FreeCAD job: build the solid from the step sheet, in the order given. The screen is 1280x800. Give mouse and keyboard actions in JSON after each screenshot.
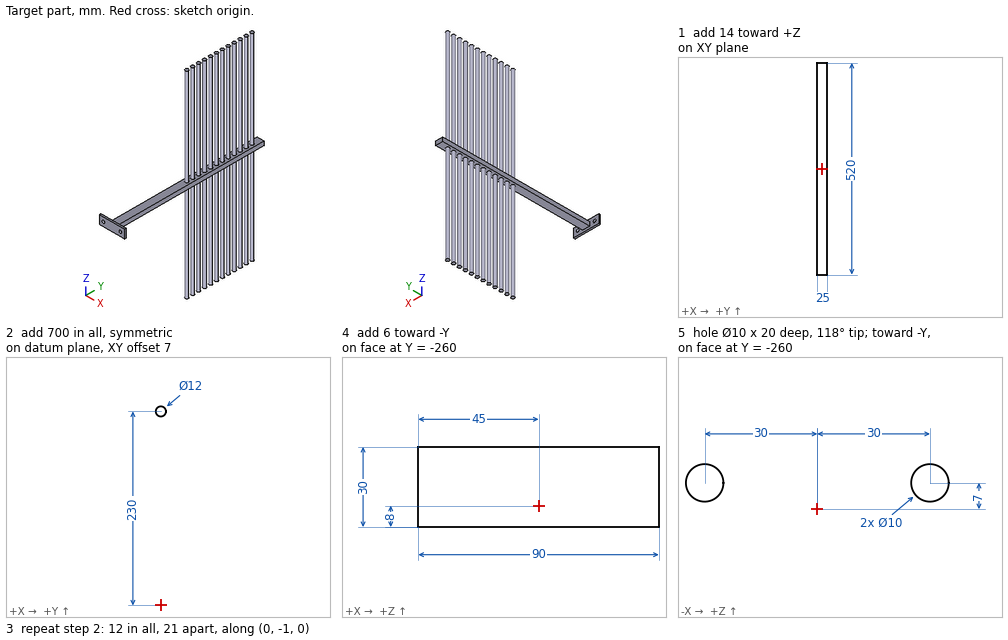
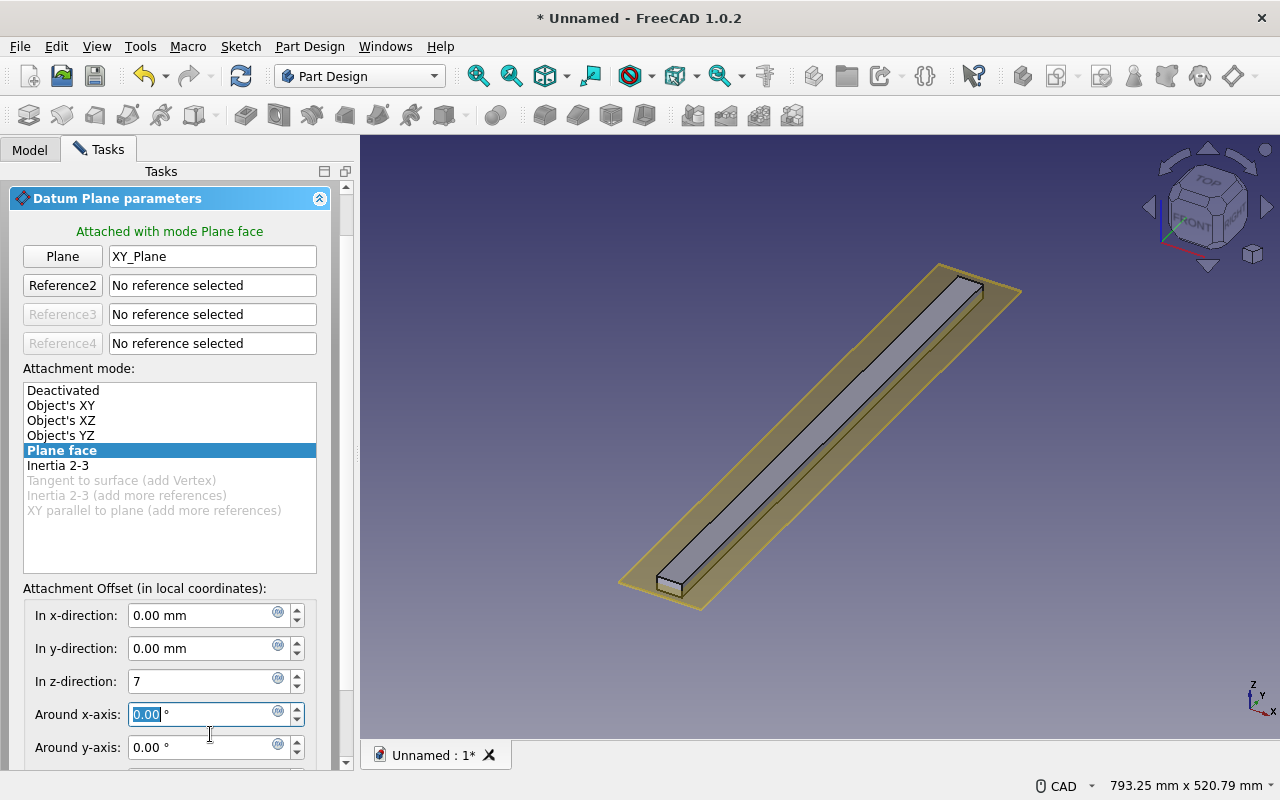
{"action": "scroll", "coordinate": [346, 476], "scroll_direction": "up", "scroll_amount": 2}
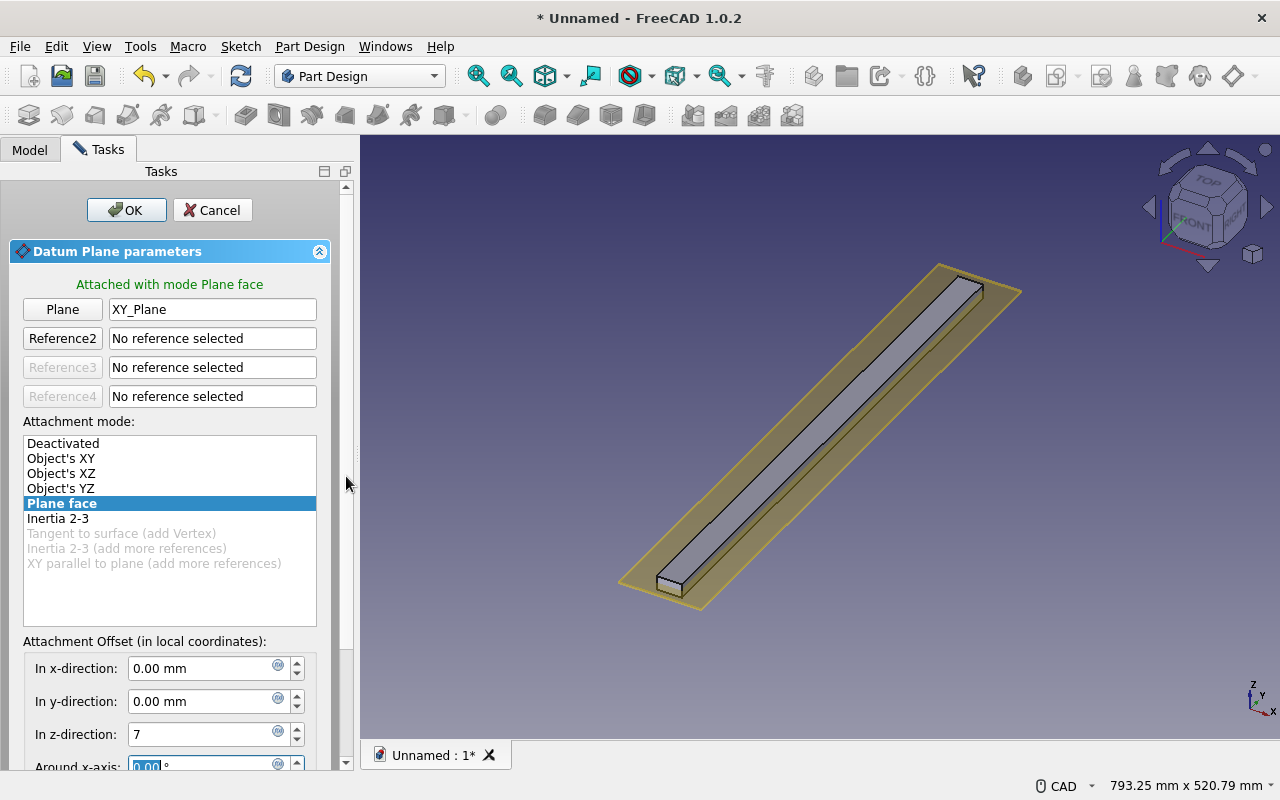
{"action": "left_click", "coordinate": [127, 210]}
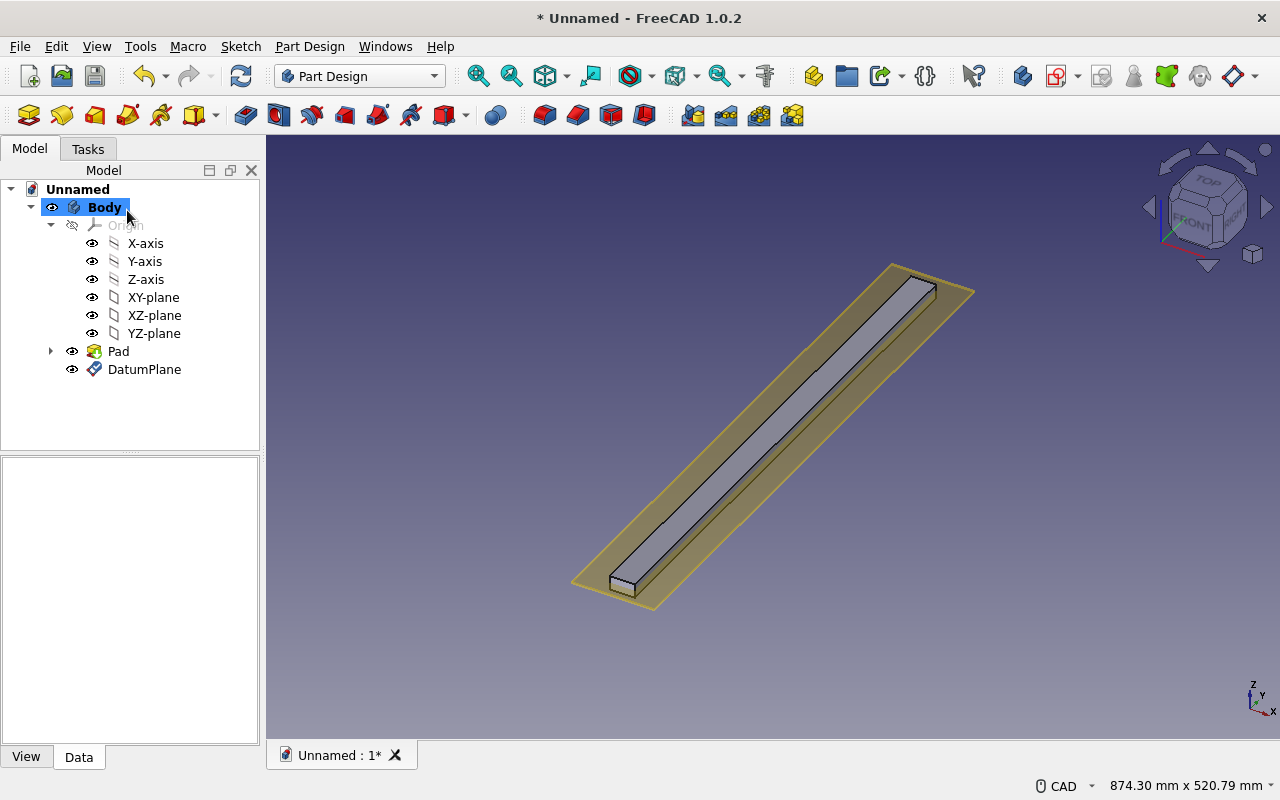
{"action": "left_click", "coordinate": [117, 369]}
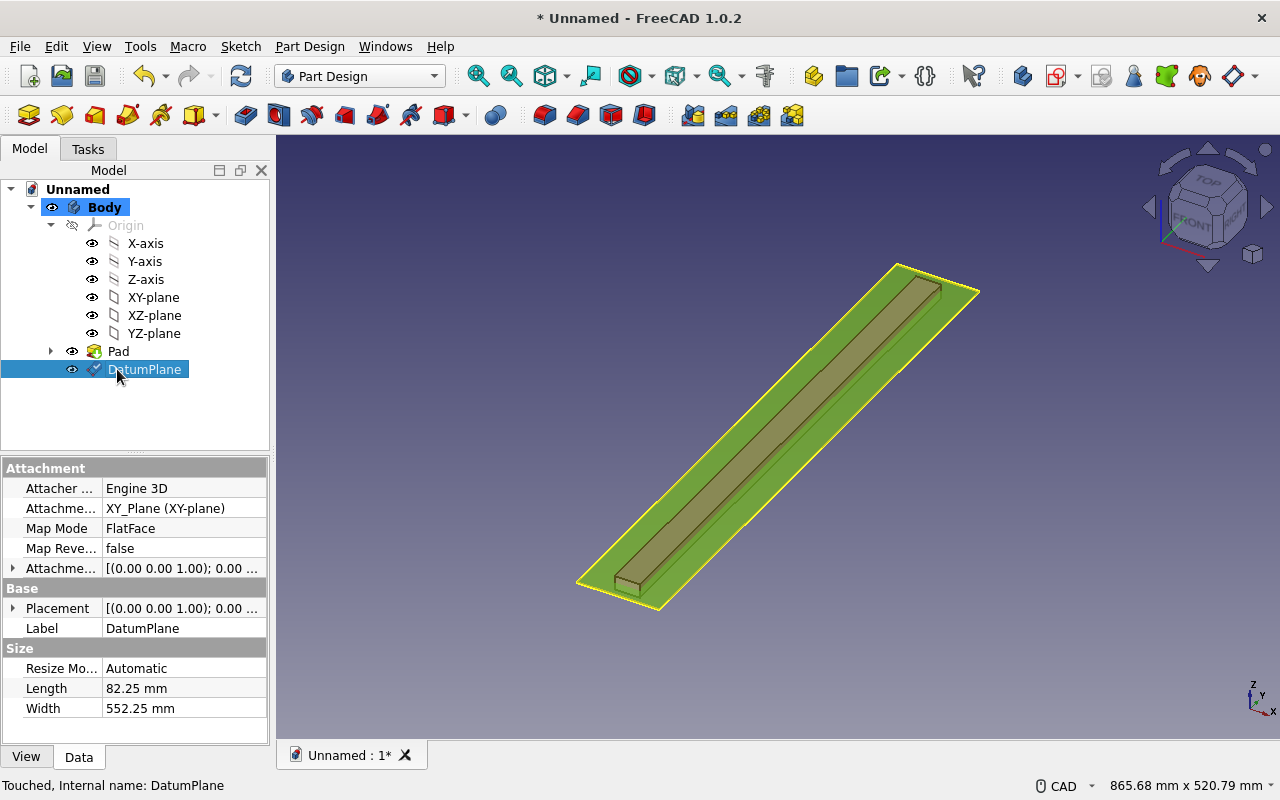
{"action": "left_click", "coordinate": [1056, 76]}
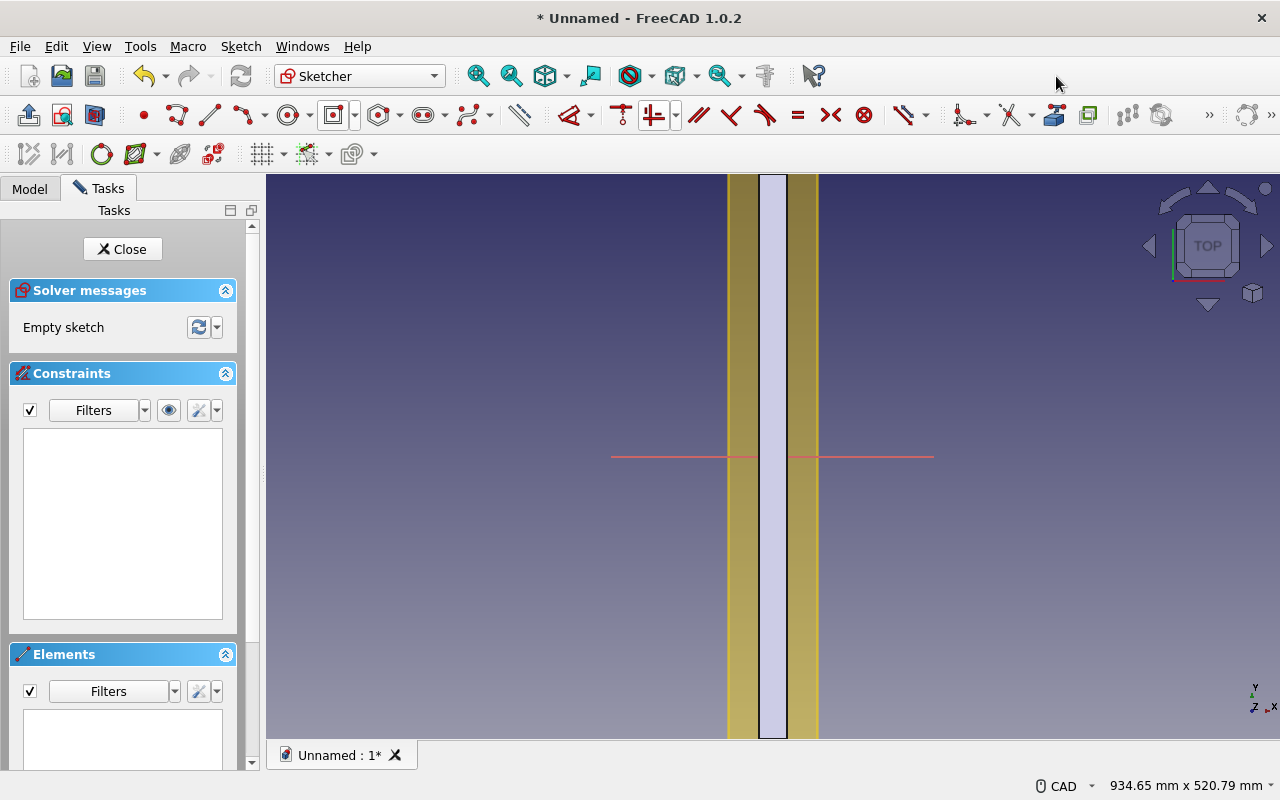
{"action": "left_click", "coordinate": [95, 116]}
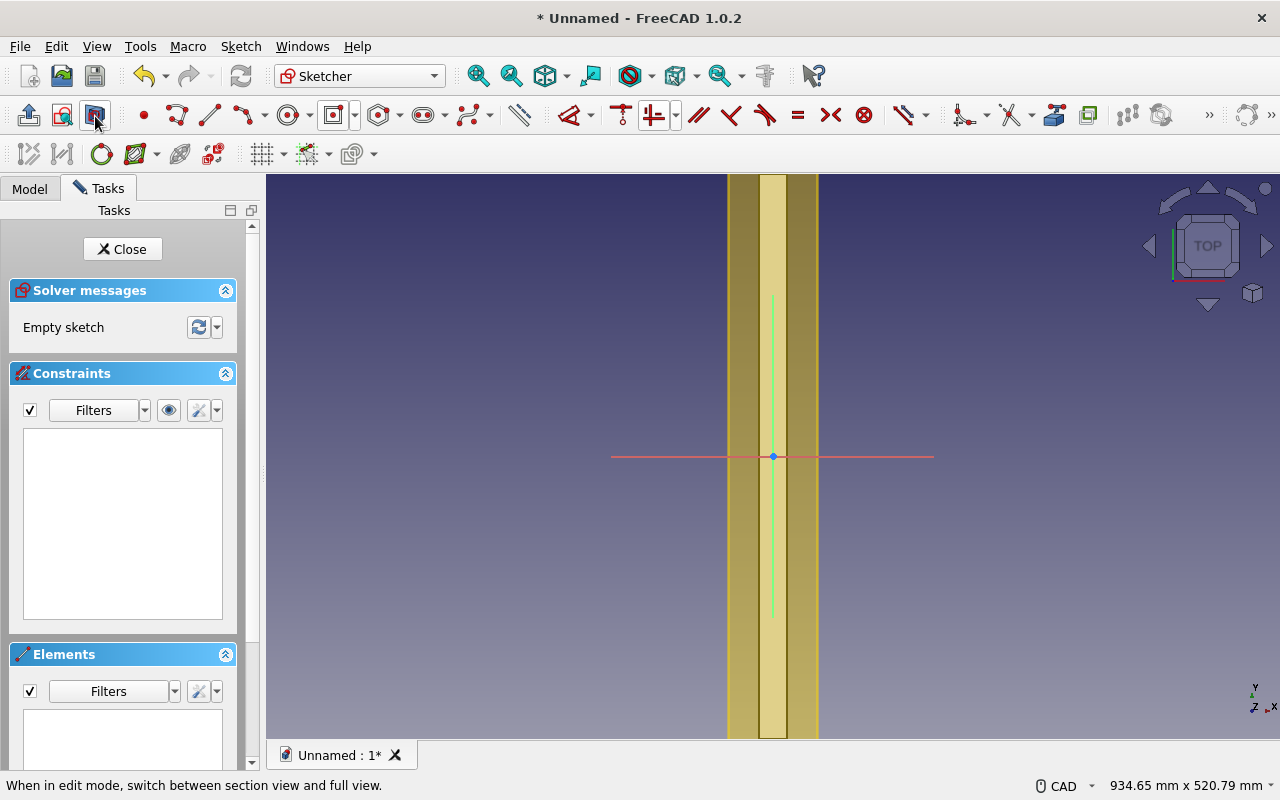
{"action": "scroll", "coordinate": [704, 456], "scroll_direction": "down", "scroll_amount": 5}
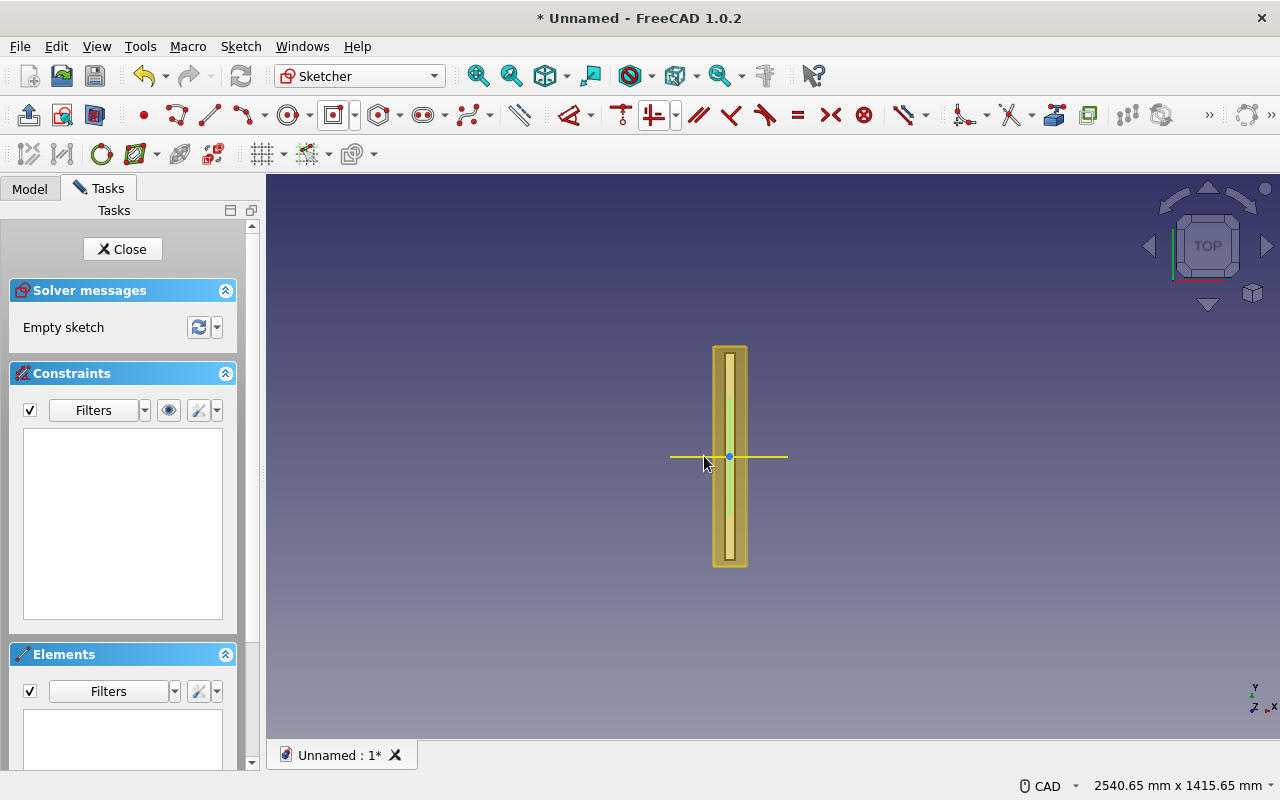
{"action": "scroll", "coordinate": [731, 360], "scroll_direction": "up", "scroll_amount": 15}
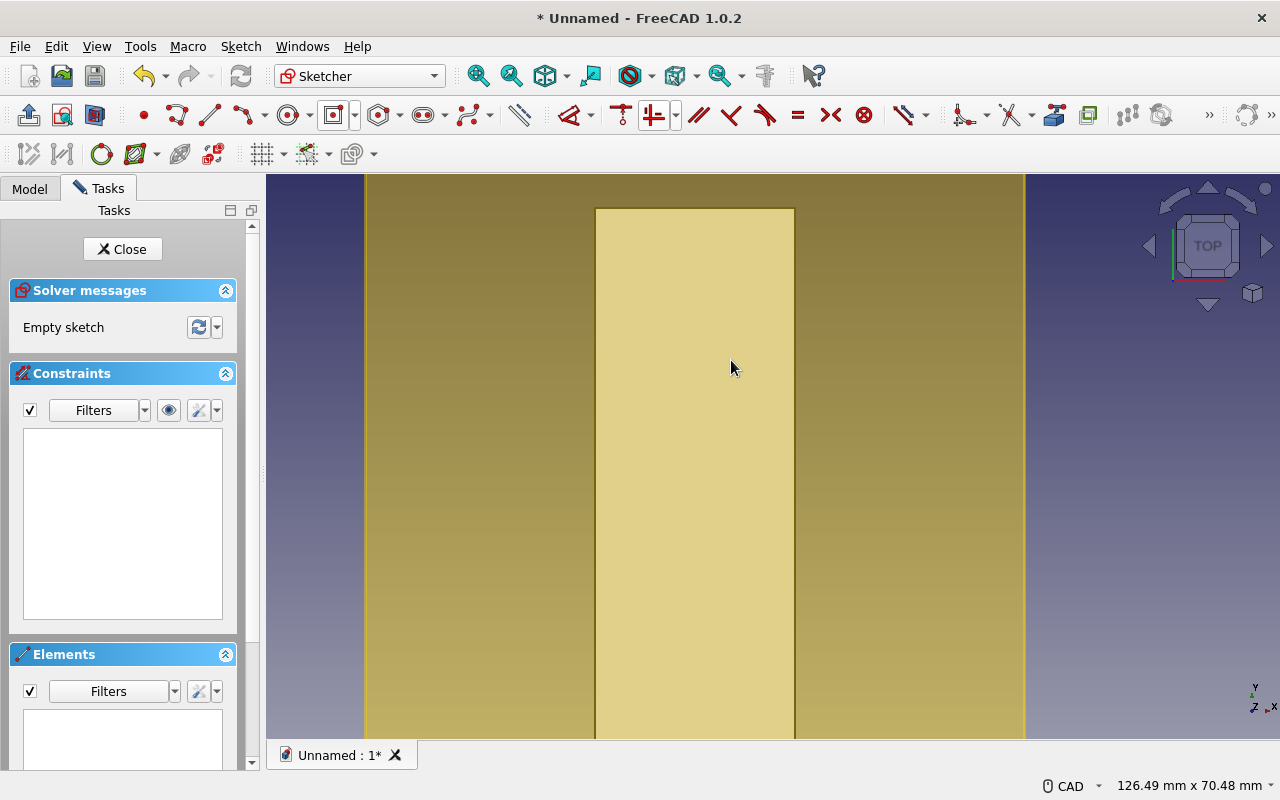
{"action": "scroll", "coordinate": [692, 445], "scroll_direction": "up", "scroll_amount": 7}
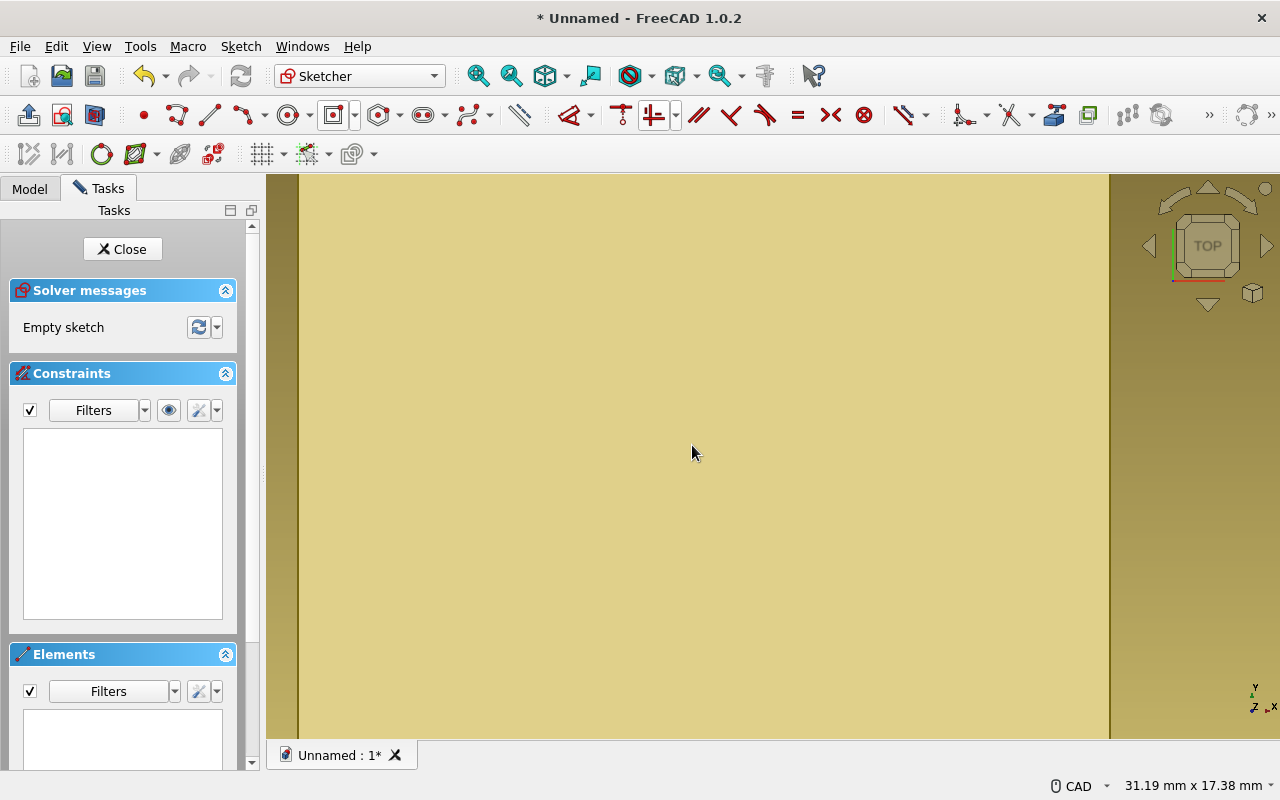
{"action": "left_click", "coordinate": [288, 116]}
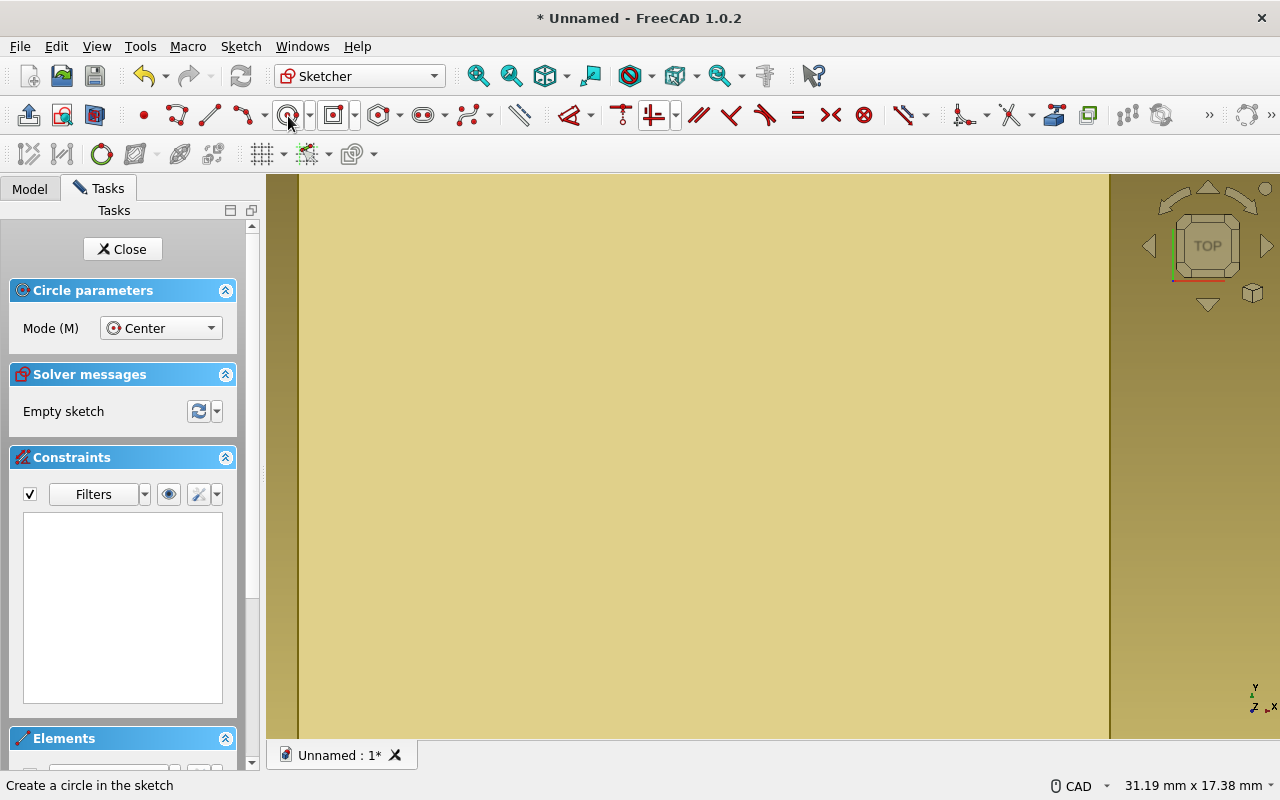
{"action": "left_click", "coordinate": [704, 457]}
{"action": "left_click", "coordinate": [842, 319]}
{"action": "key", "text": "Escape"}